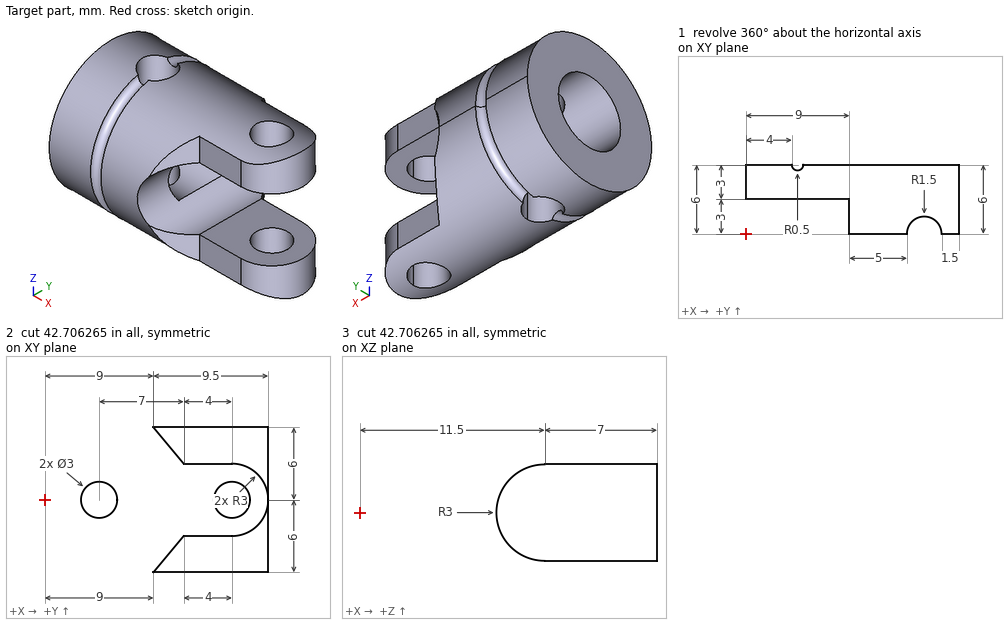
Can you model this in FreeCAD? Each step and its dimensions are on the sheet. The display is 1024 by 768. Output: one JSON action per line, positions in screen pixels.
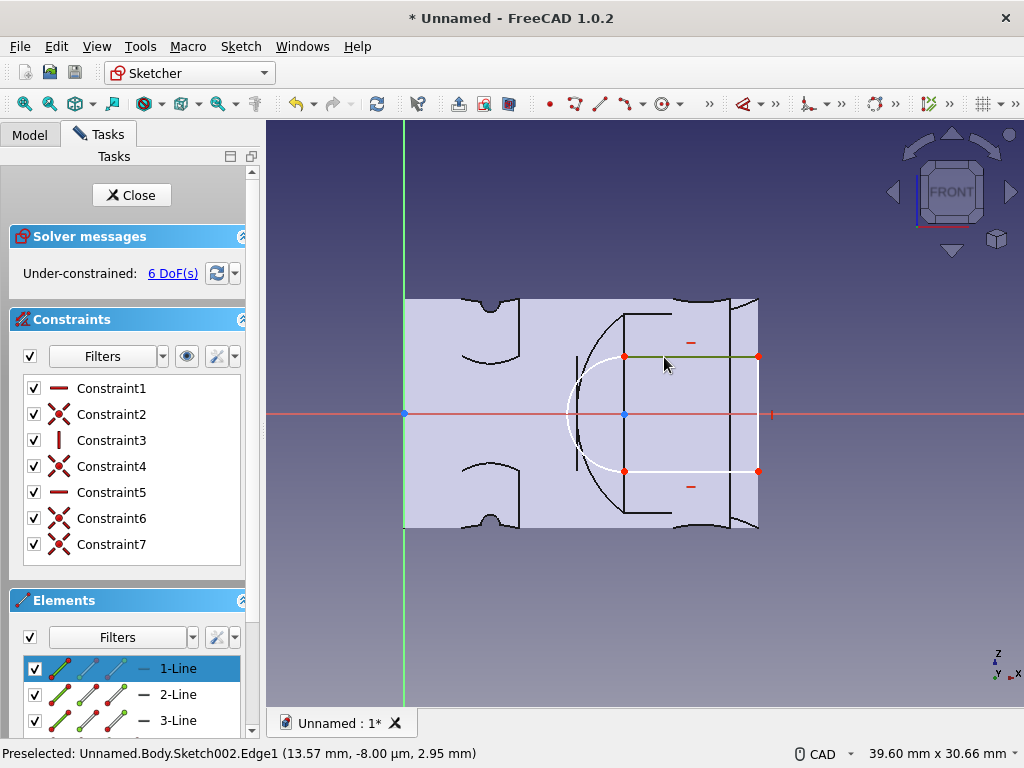
{"action": "left_click", "coordinate": [578, 381]}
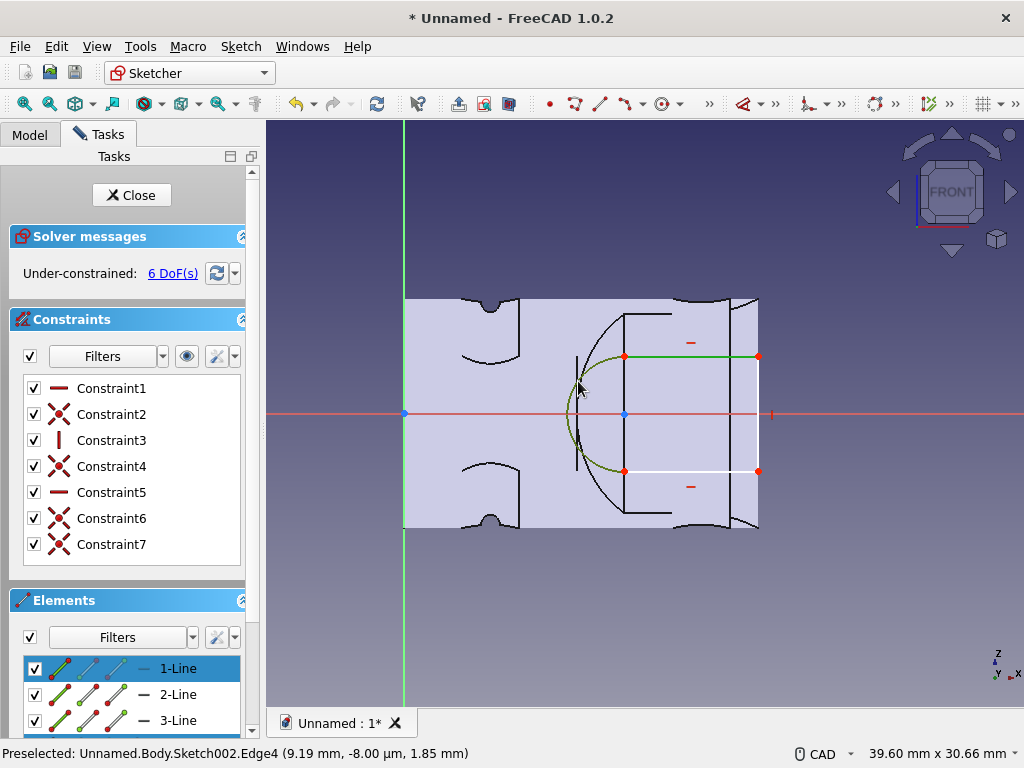
{"action": "key", "text": "t"}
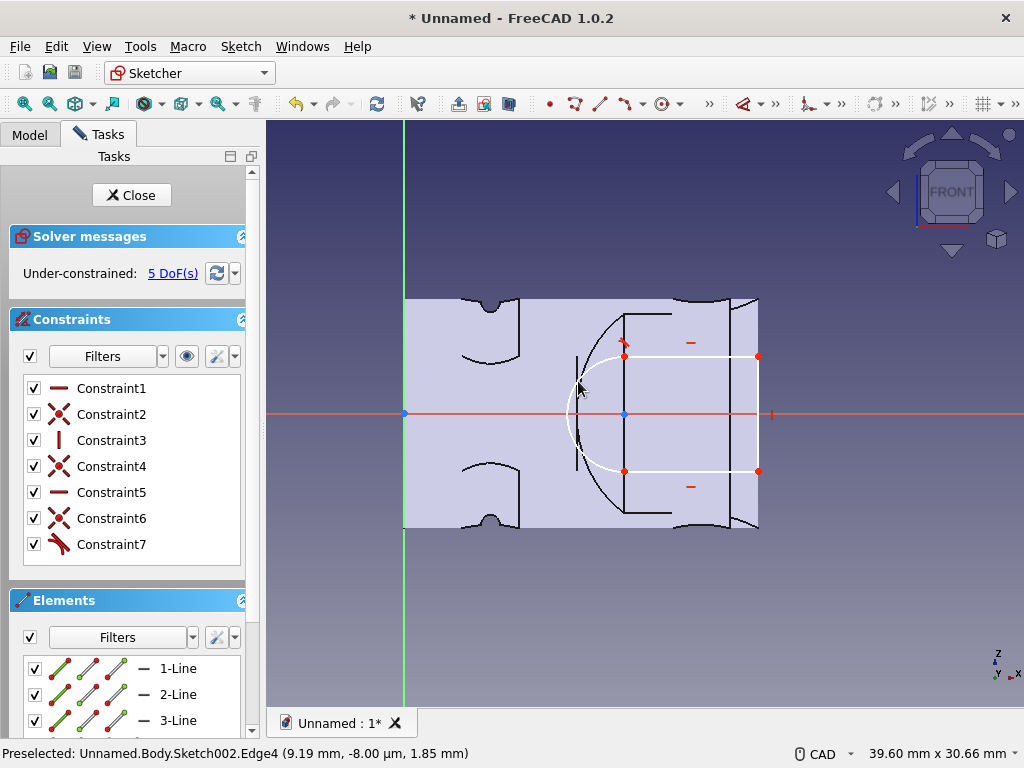
{"action": "left_click", "coordinate": [718, 472]}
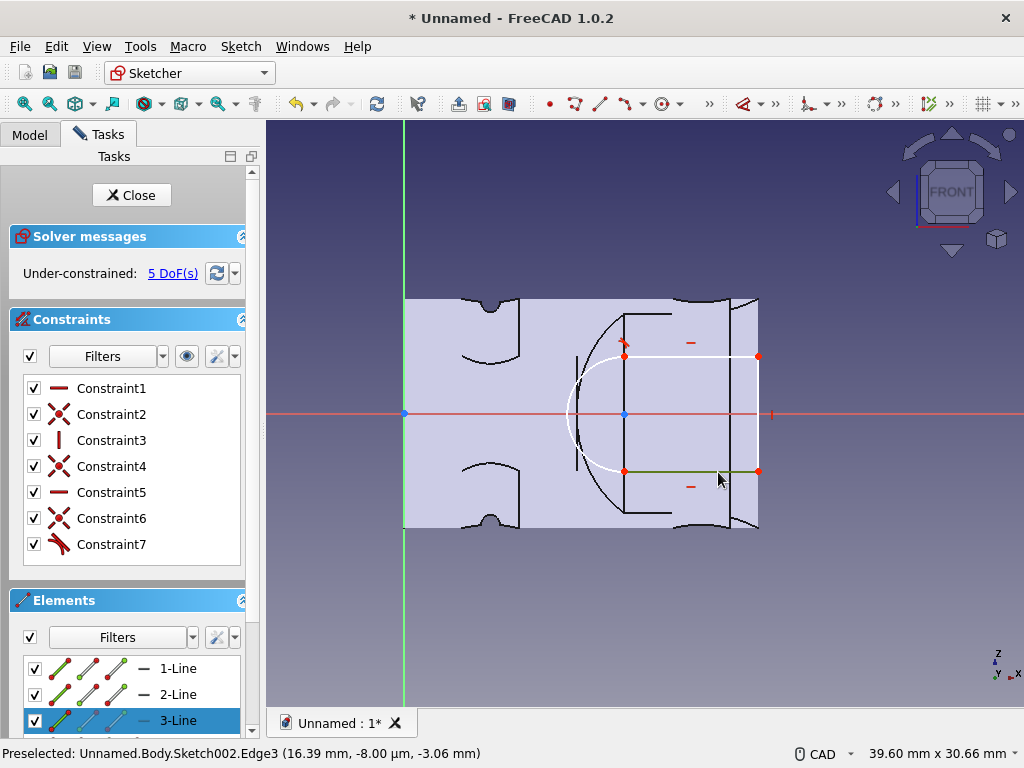
{"action": "left_click", "coordinate": [578, 381]}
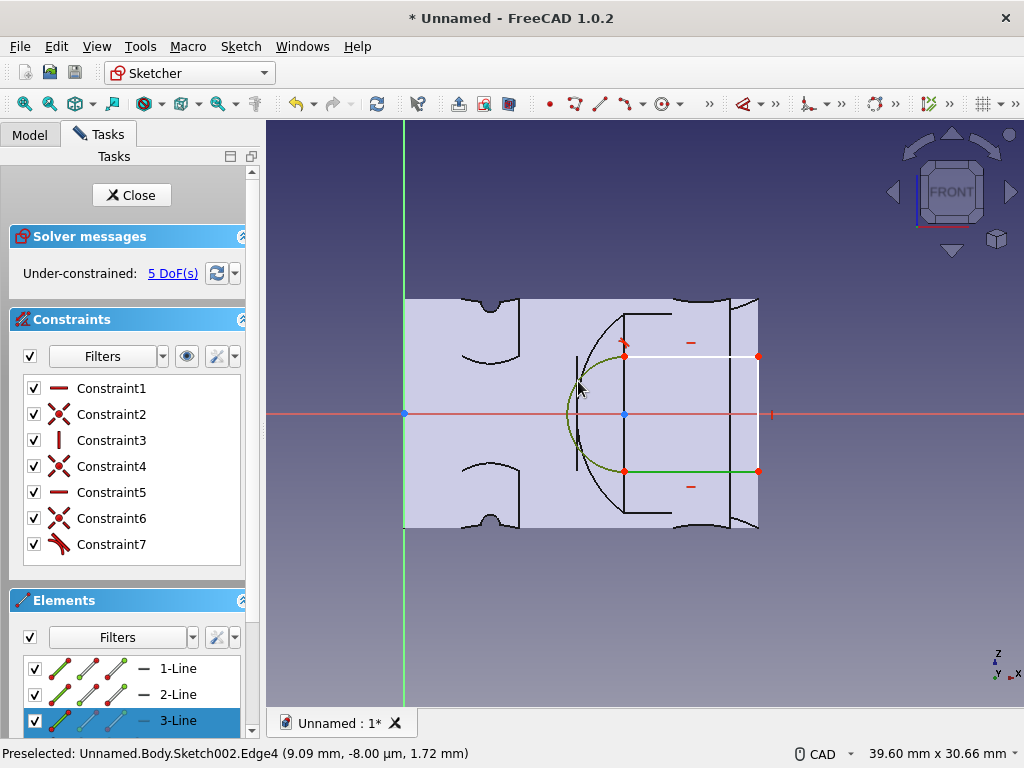
{"action": "key", "text": "t"}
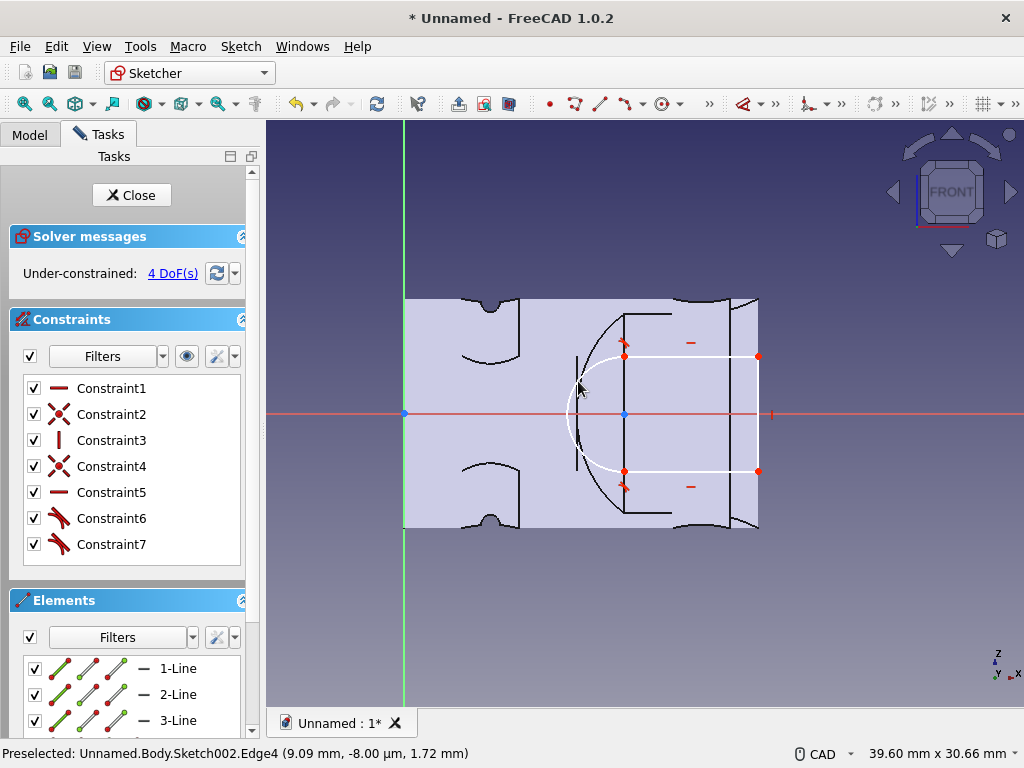
{"action": "left_click", "coordinate": [625, 414]}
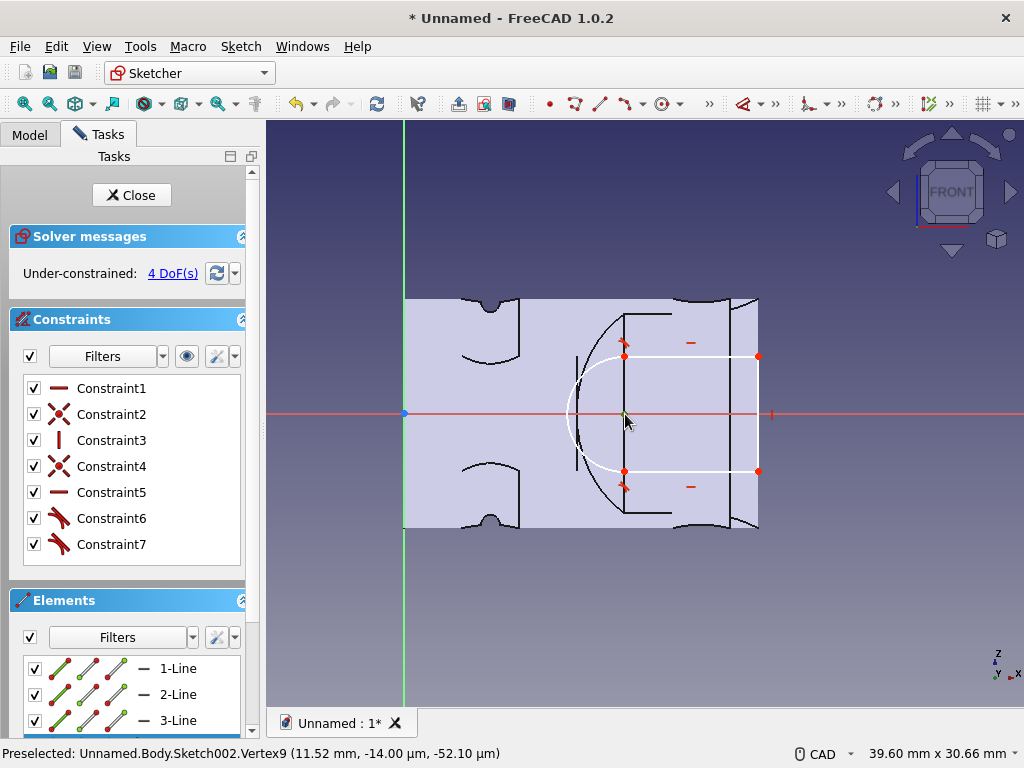
{"action": "left_click", "coordinate": [334, 414]}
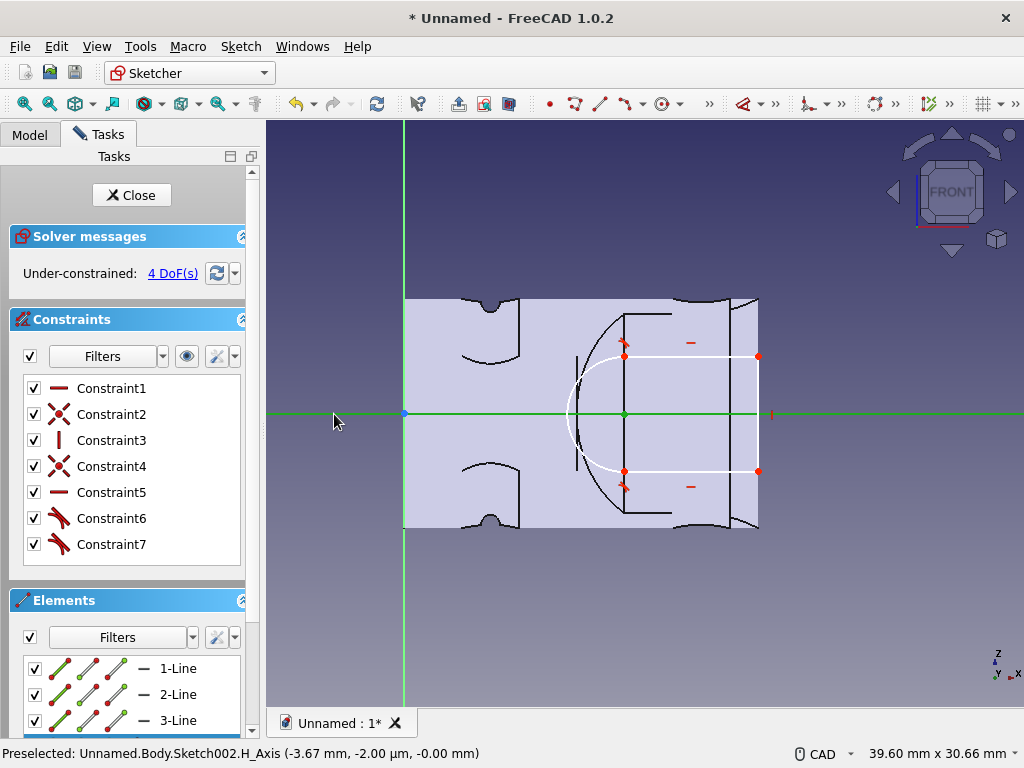
{"action": "key", "text": "c"}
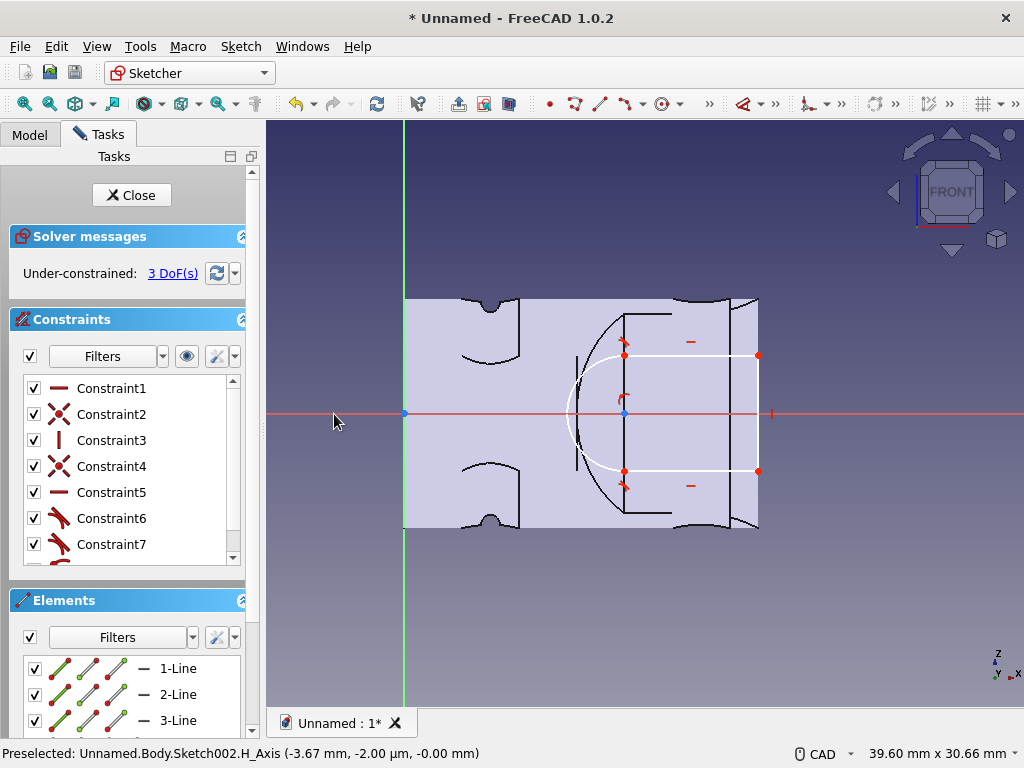
{"action": "left_click", "coordinate": [742, 104]}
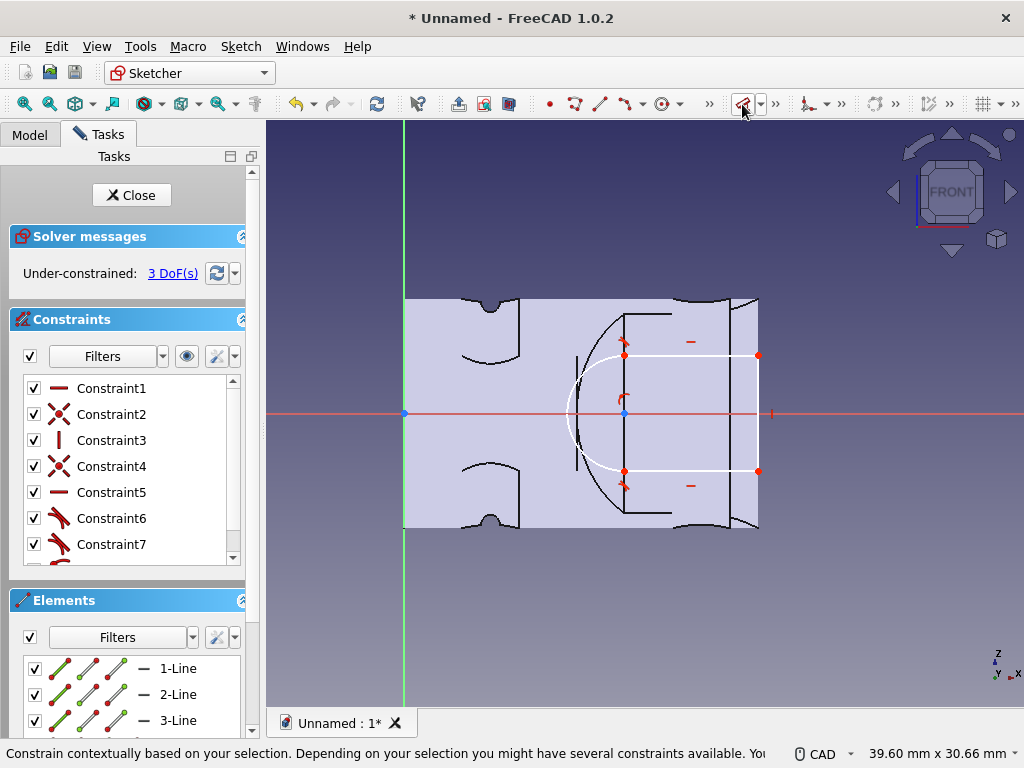
{"action": "left_click", "coordinate": [578, 380]}
{"action": "left_click", "coordinate": [552, 361]}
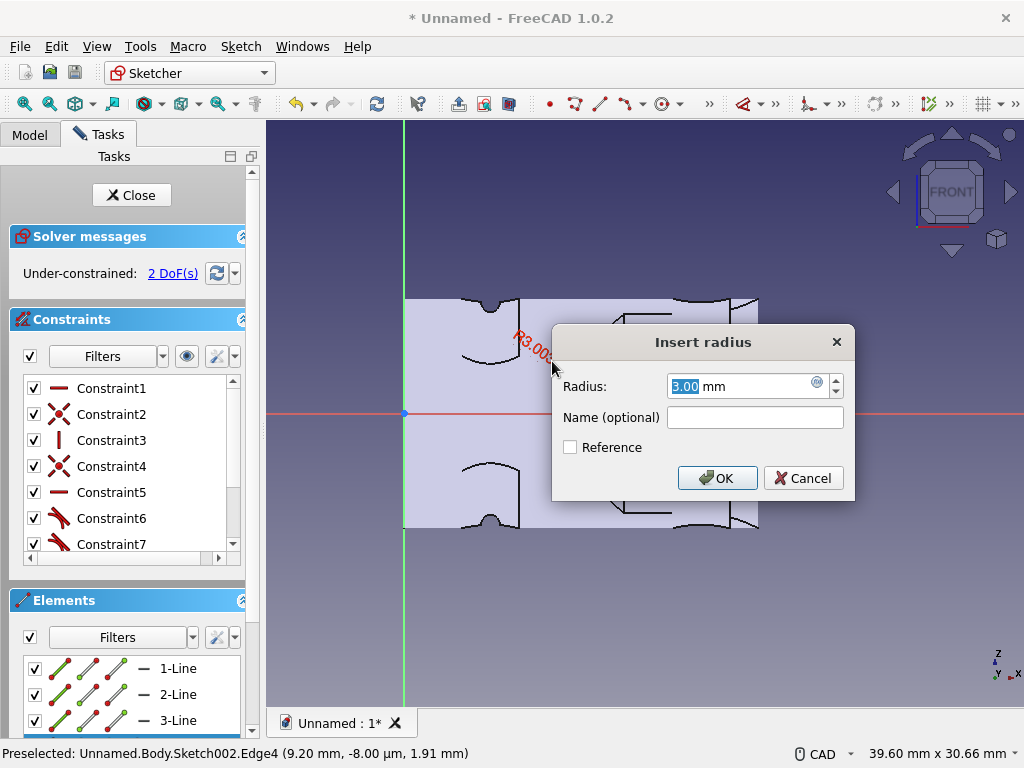
{"action": "type", "text": "3"}
{"action": "key", "text": "Return"}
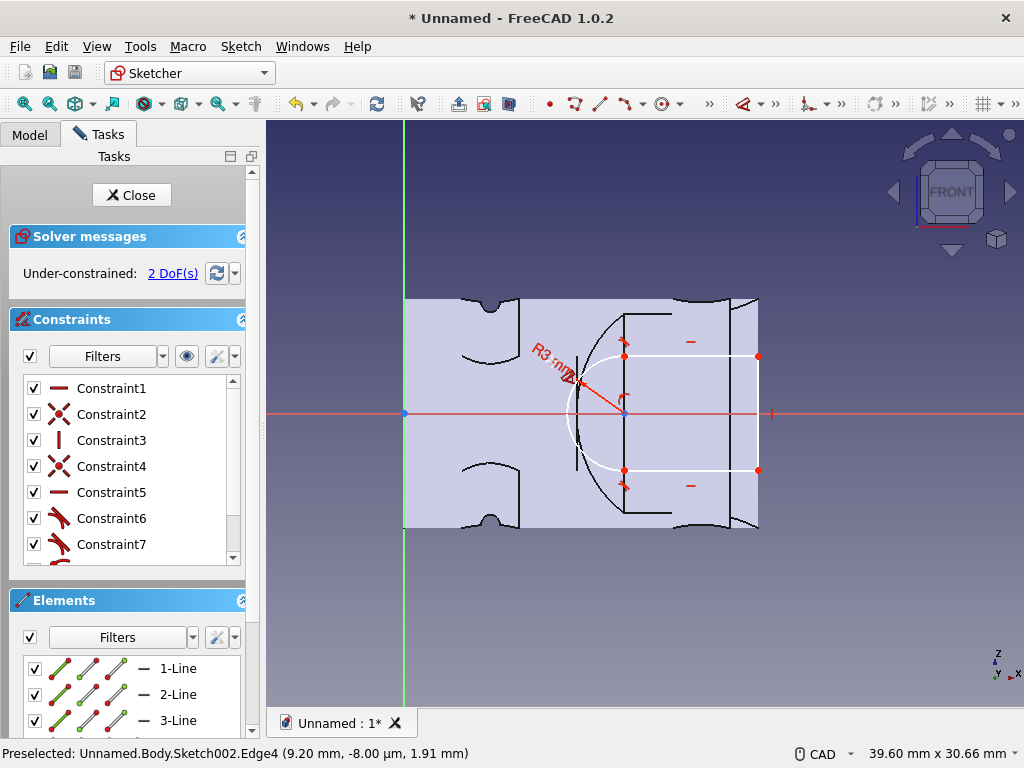
{"action": "left_click", "coordinate": [665, 356]}
{"action": "left_click", "coordinate": [691, 322]}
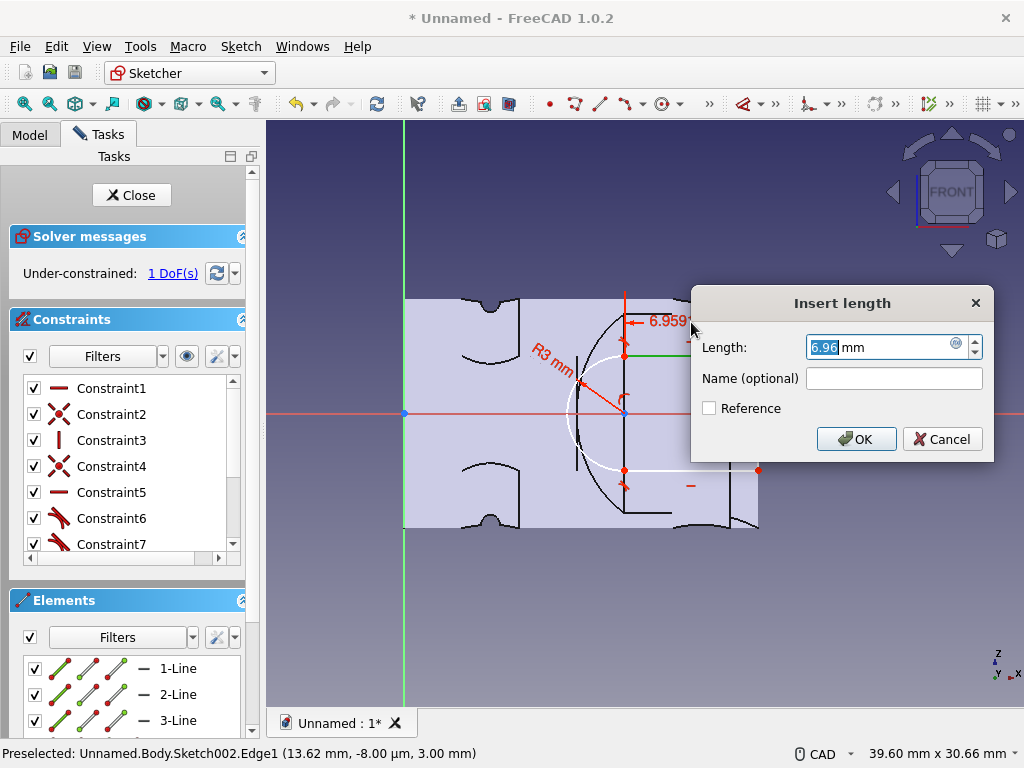
{"action": "type", "text": "7"}
{"action": "key", "text": "Return"}